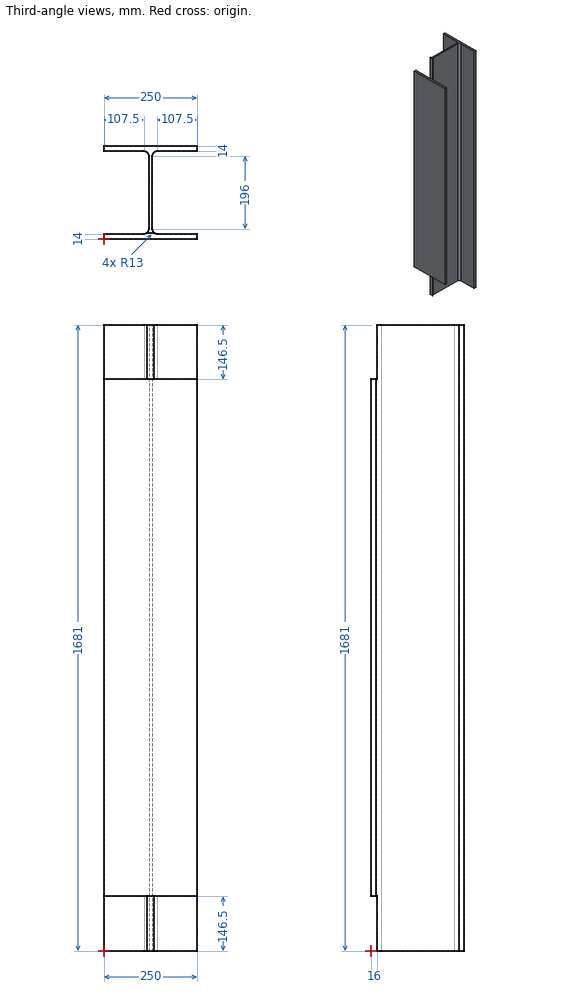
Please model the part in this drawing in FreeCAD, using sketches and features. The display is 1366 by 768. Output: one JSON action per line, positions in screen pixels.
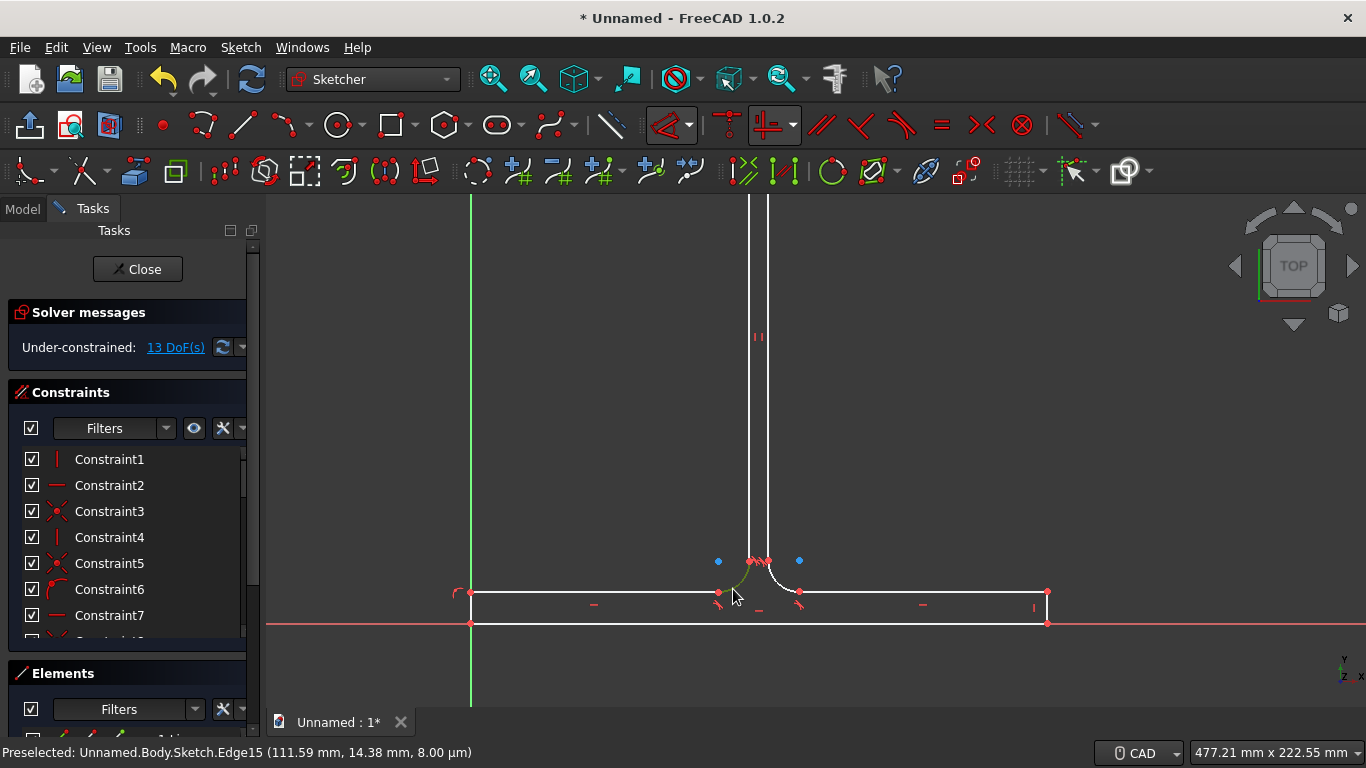
{"action": "left_click", "coordinate": [772, 575]}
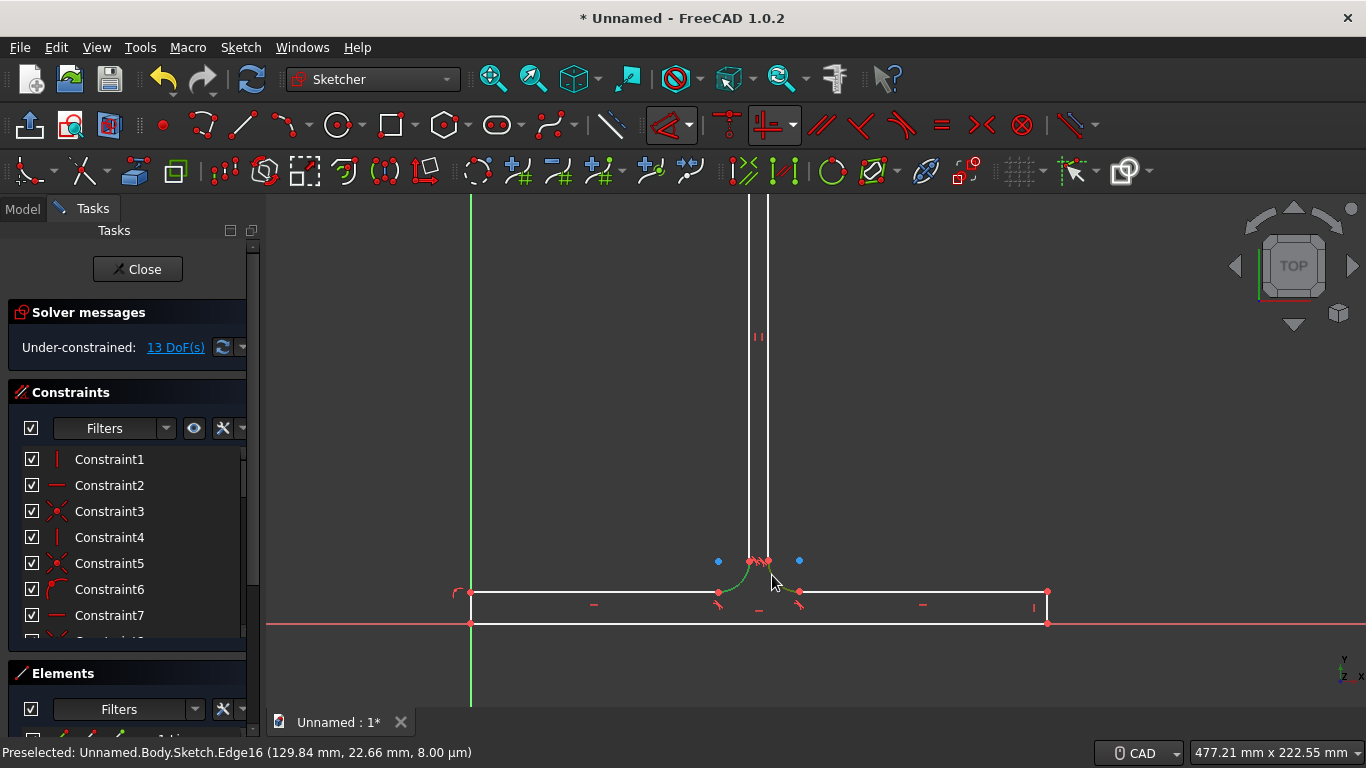
{"action": "left_click", "coordinate": [942, 126]}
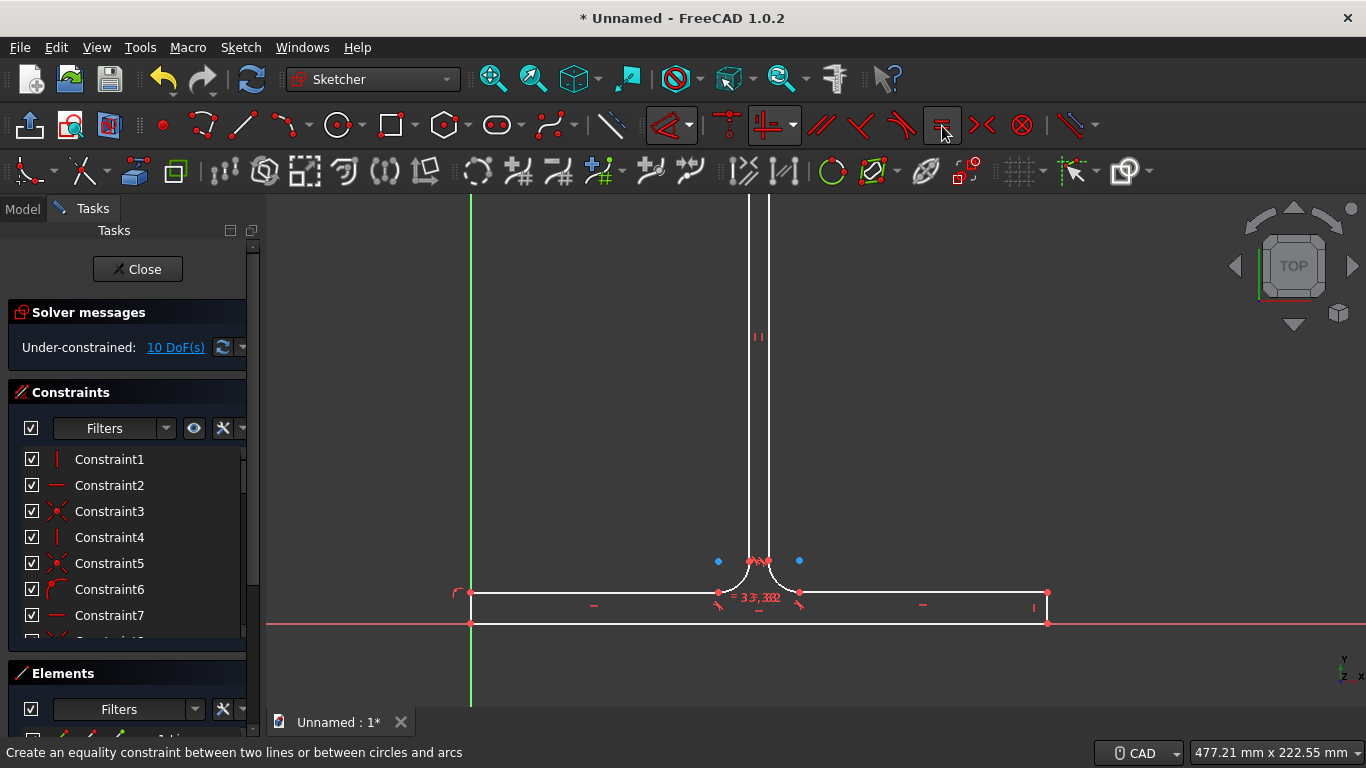
{"action": "scroll", "coordinate": [733, 590], "scroll_direction": "down", "scroll_amount": 3}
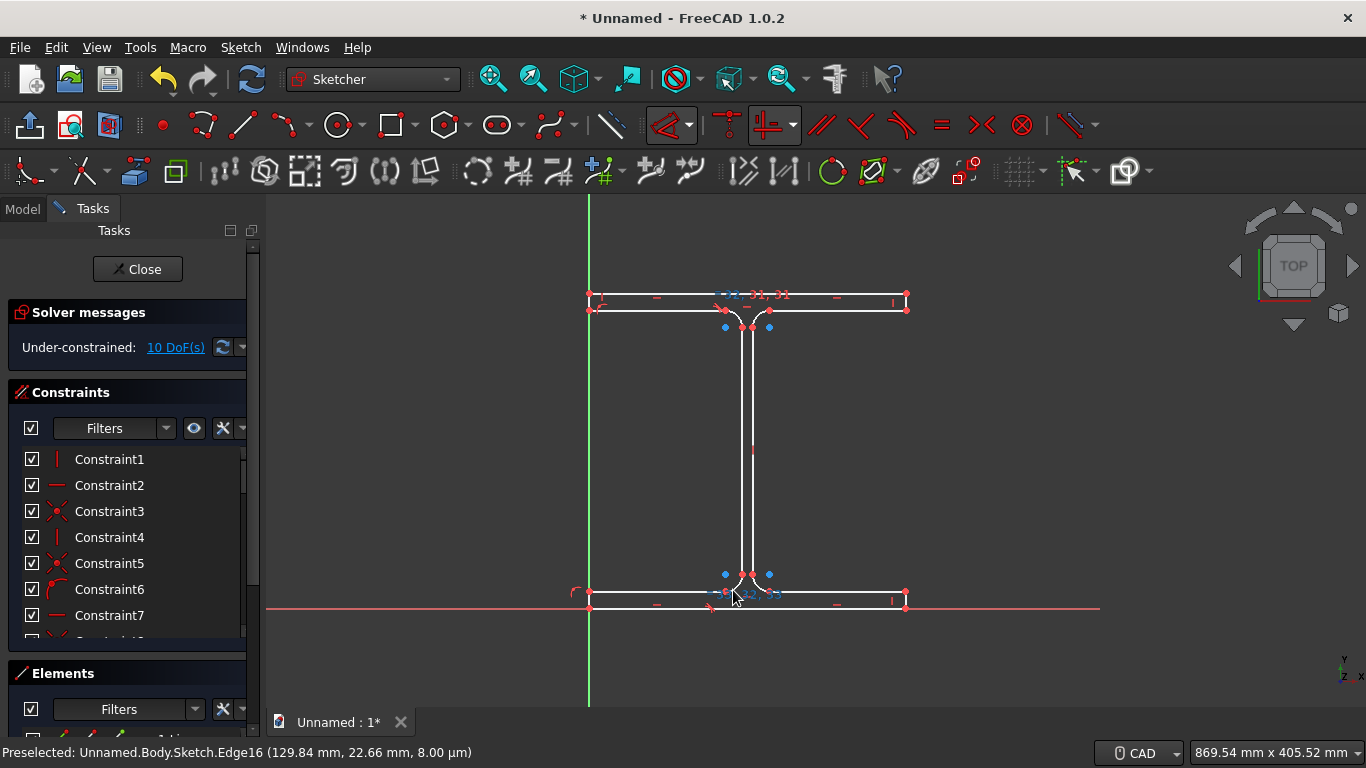
{"action": "scroll", "coordinate": [762, 313], "scroll_direction": "up", "scroll_amount": 5}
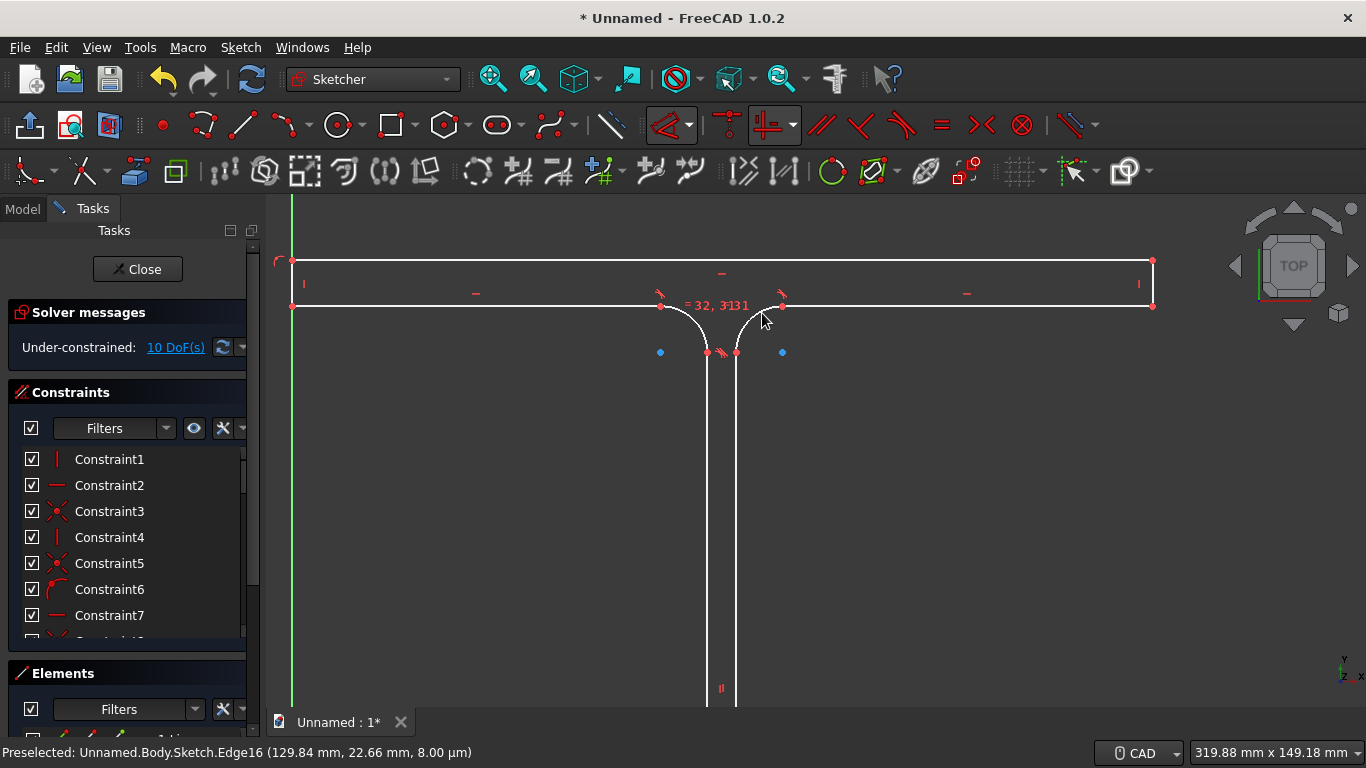
{"action": "left_click", "coordinate": [761, 311]}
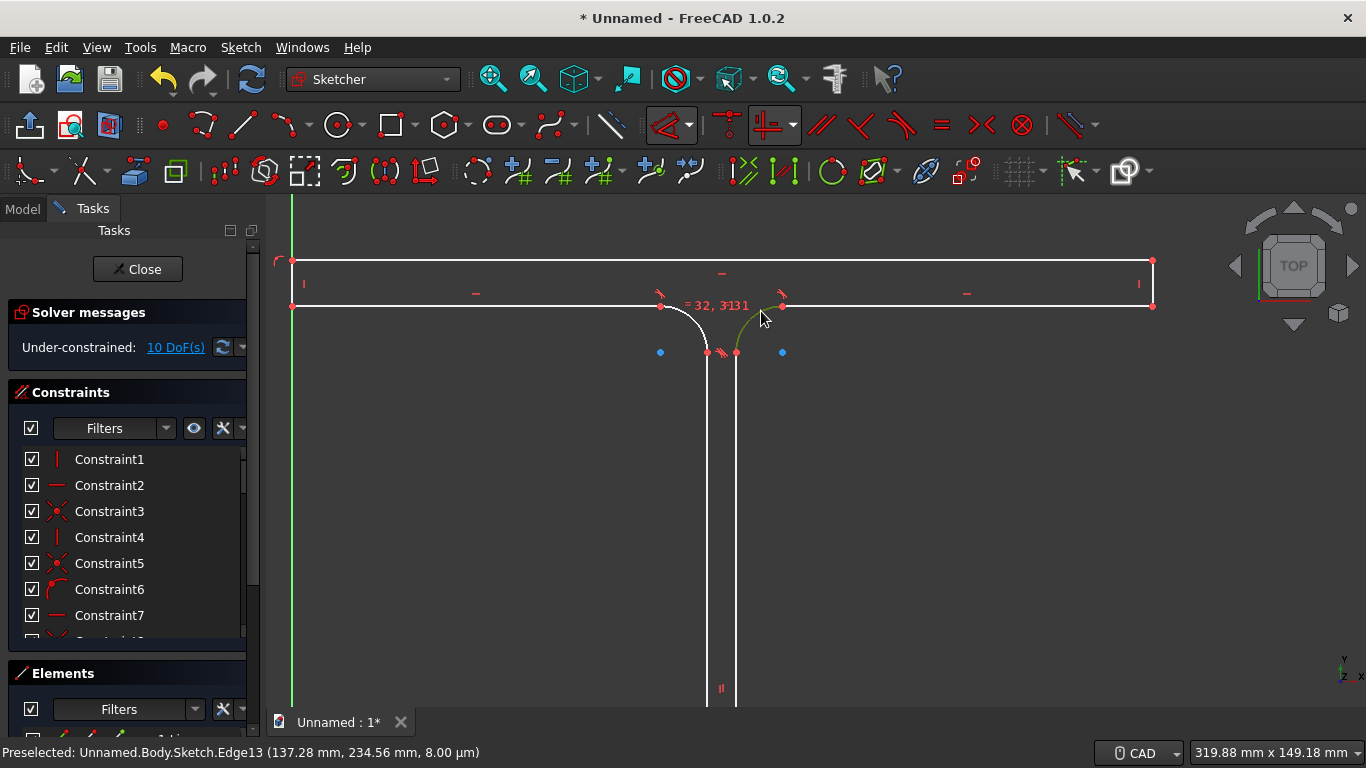
{"action": "left_click", "coordinate": [692, 126]}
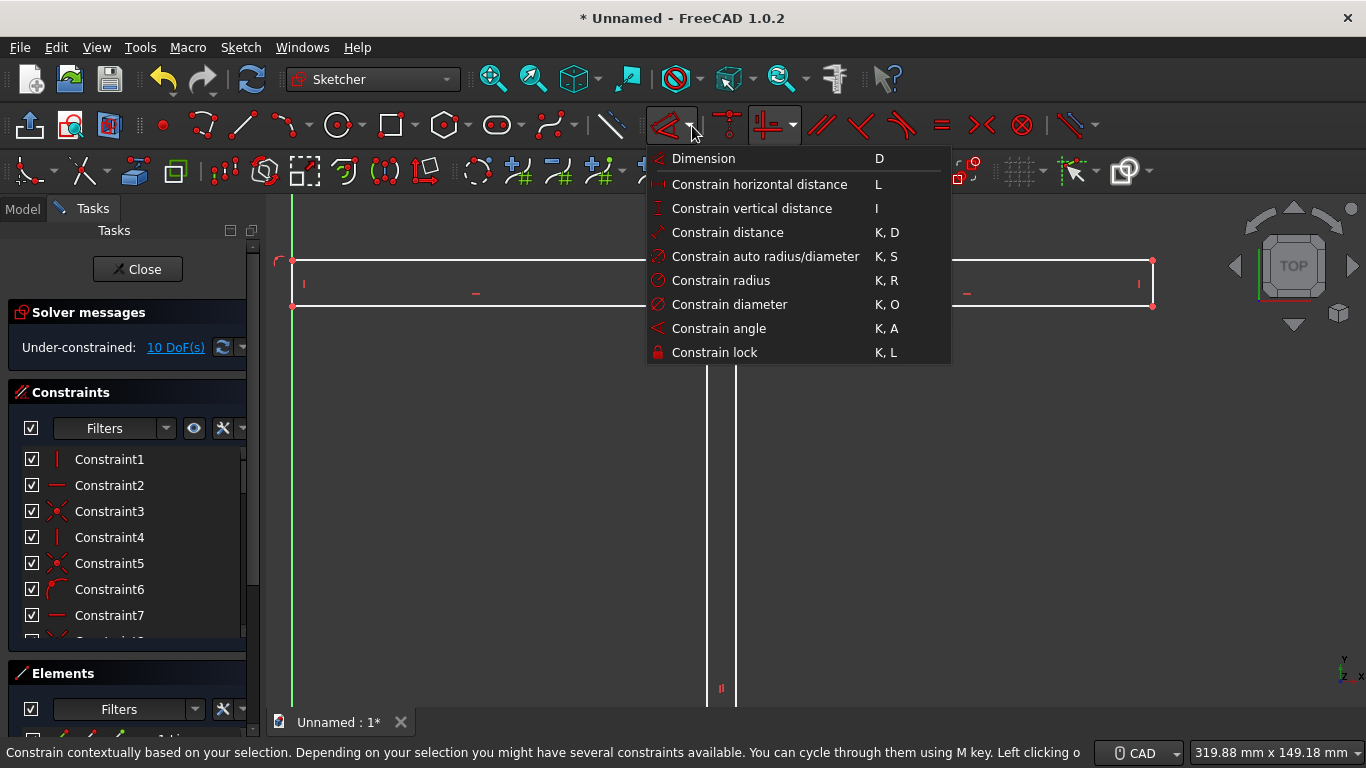
{"action": "left_click", "coordinate": [799, 280]}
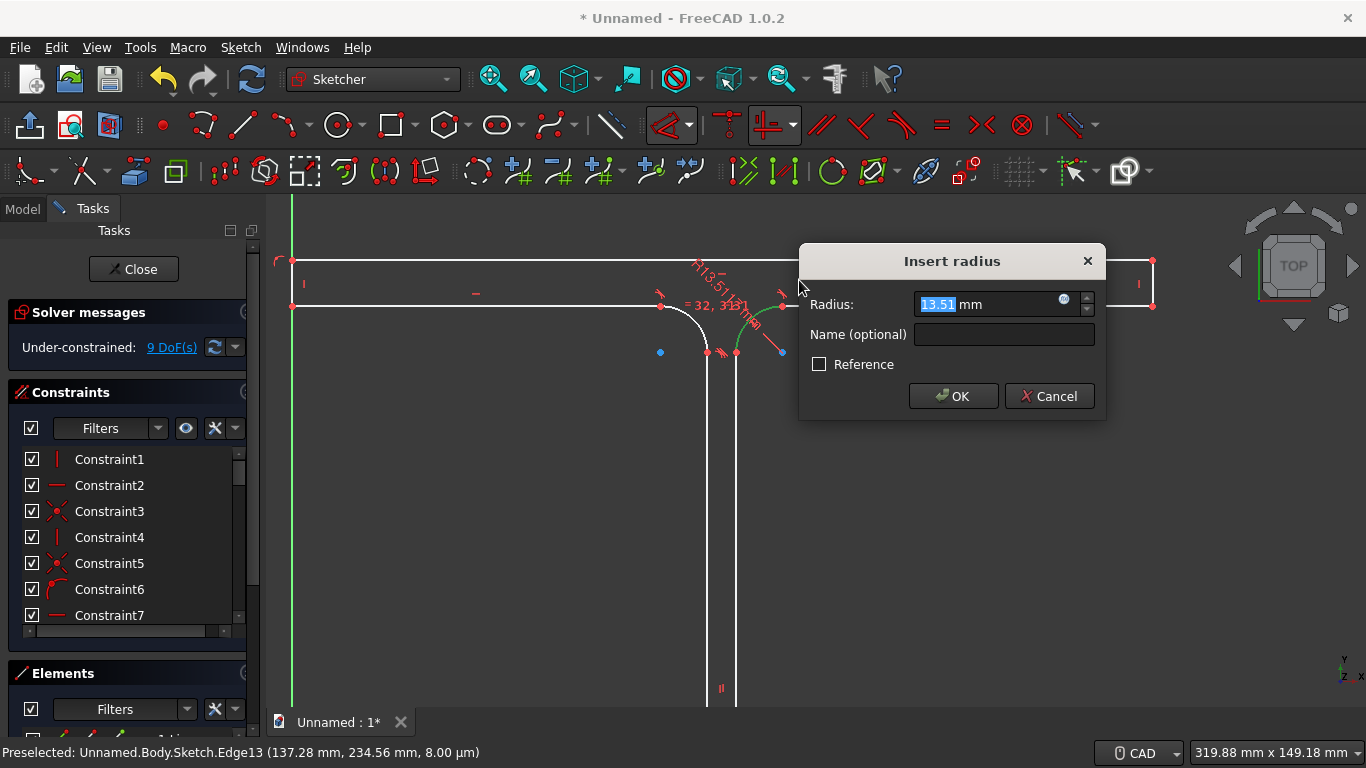
{"action": "type", "text": "13"}
{"action": "key", "text": "Return"}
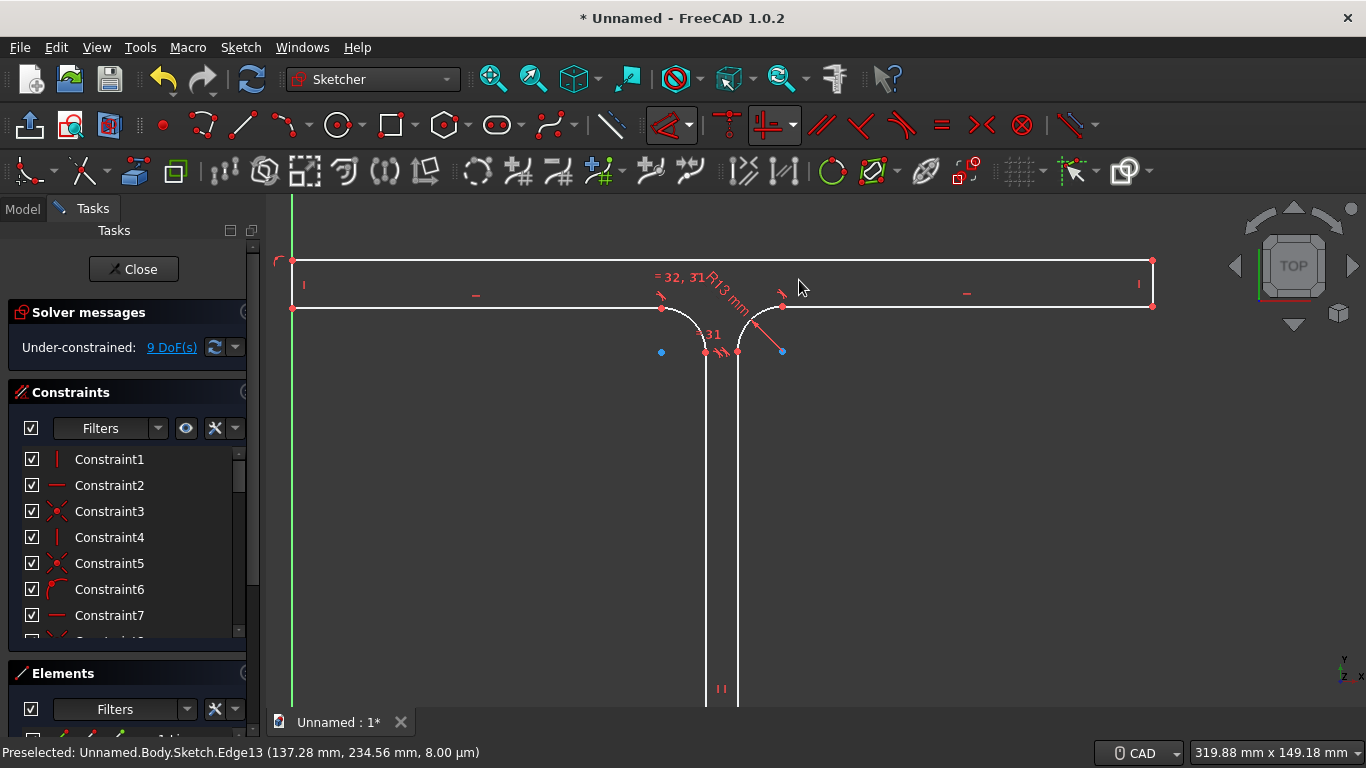
{"action": "left_click", "coordinate": [1153, 293]}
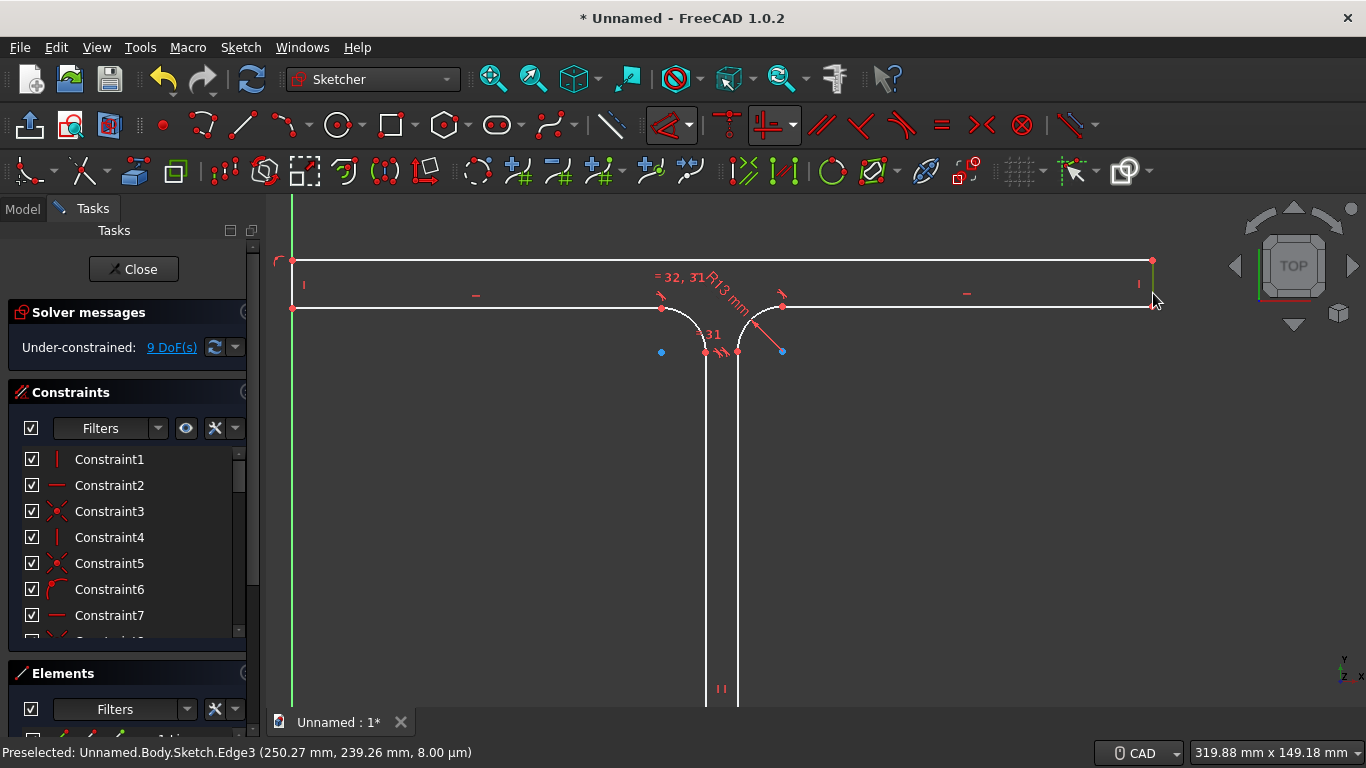
{"action": "key", "text": "i"}